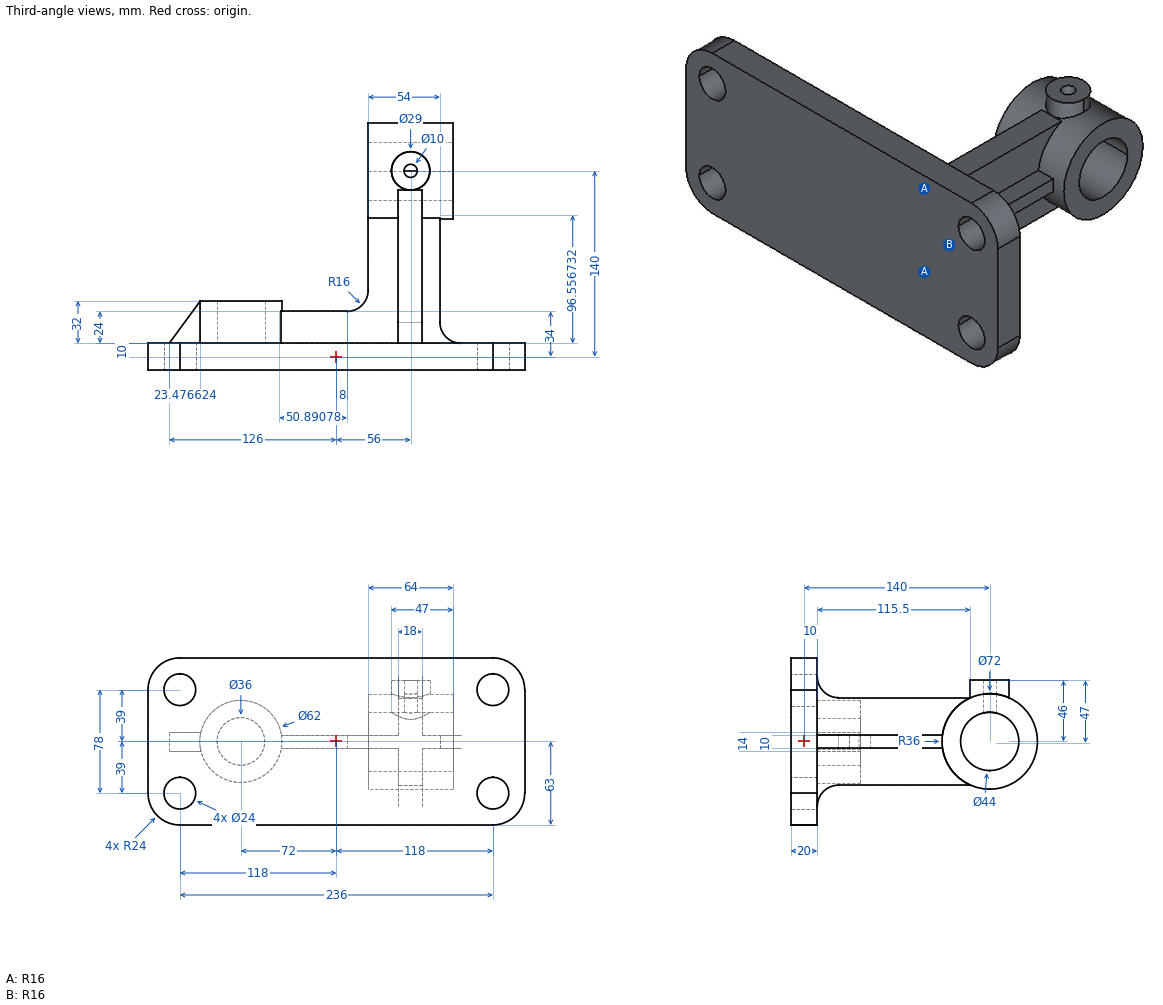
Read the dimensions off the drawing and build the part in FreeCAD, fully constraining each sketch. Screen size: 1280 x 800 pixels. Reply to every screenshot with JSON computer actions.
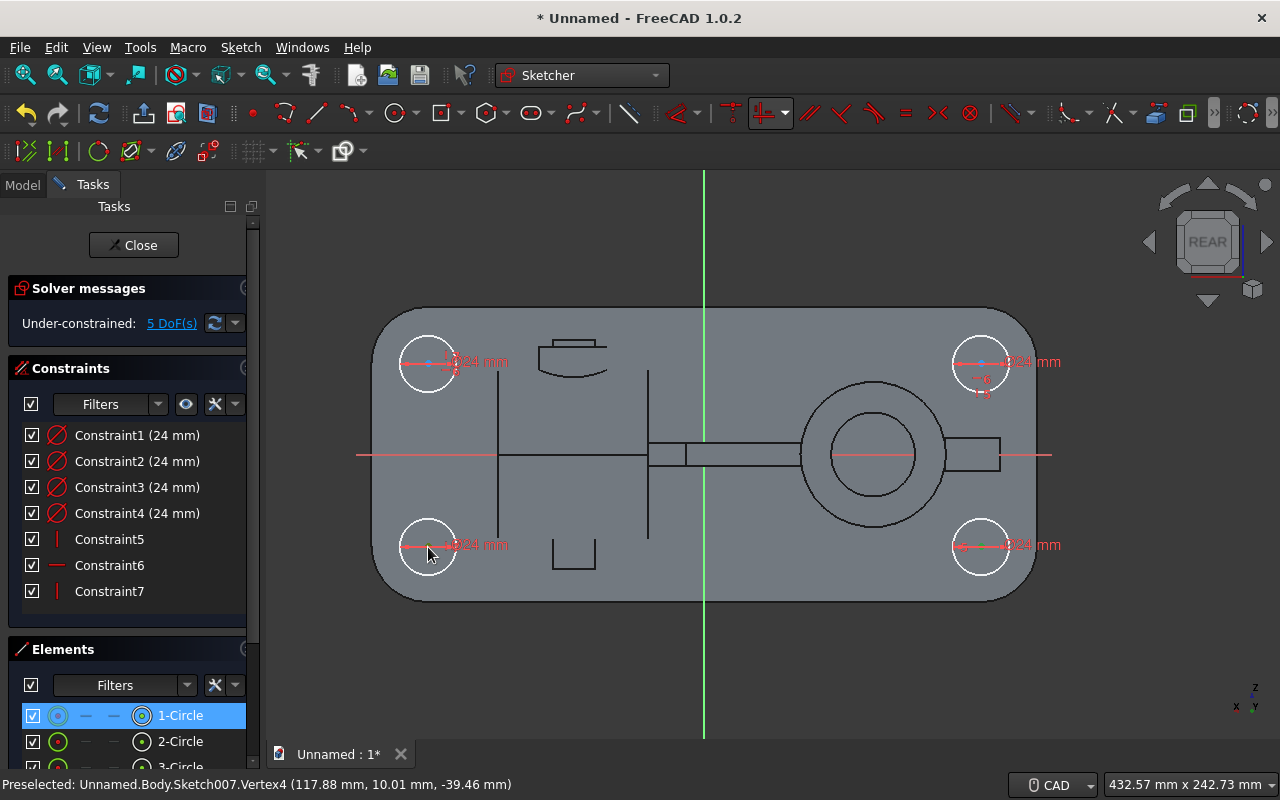
{"action": "key", "text": "h"}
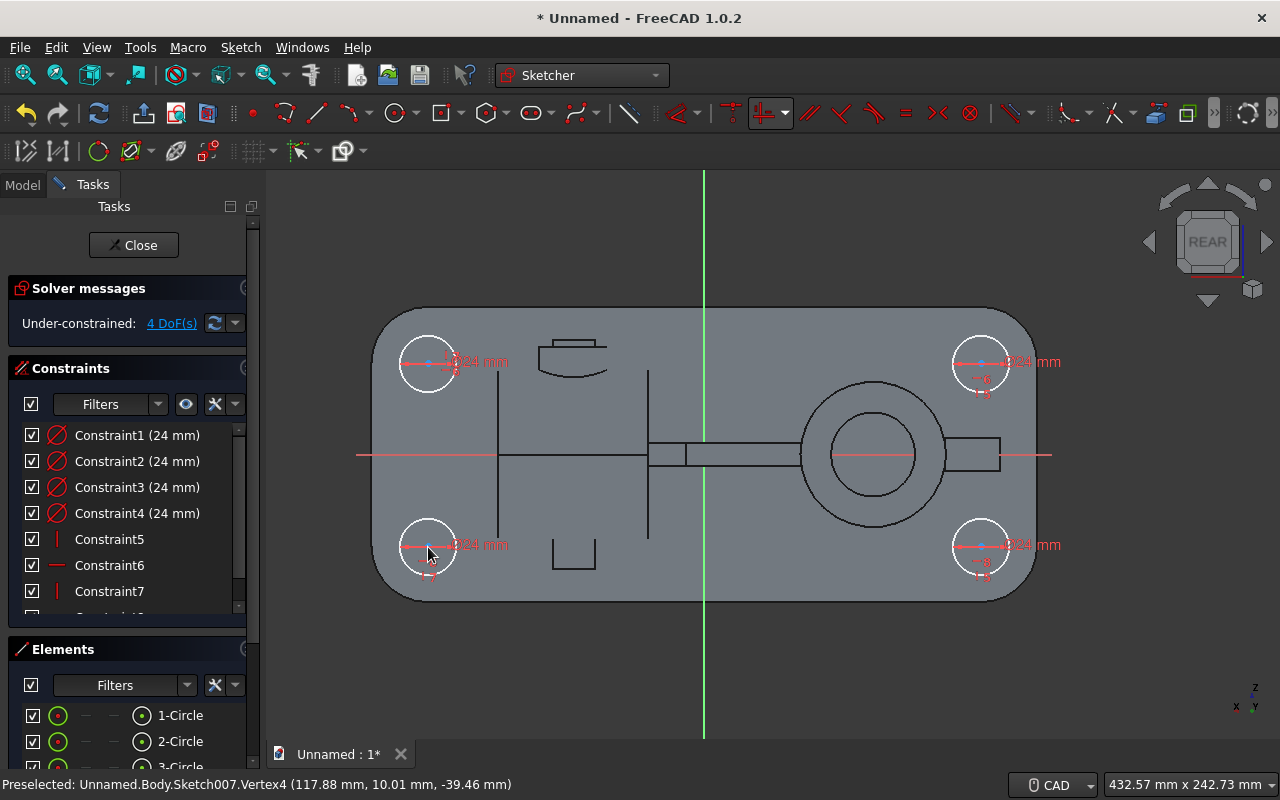
{"action": "left_click", "coordinate": [676, 114]}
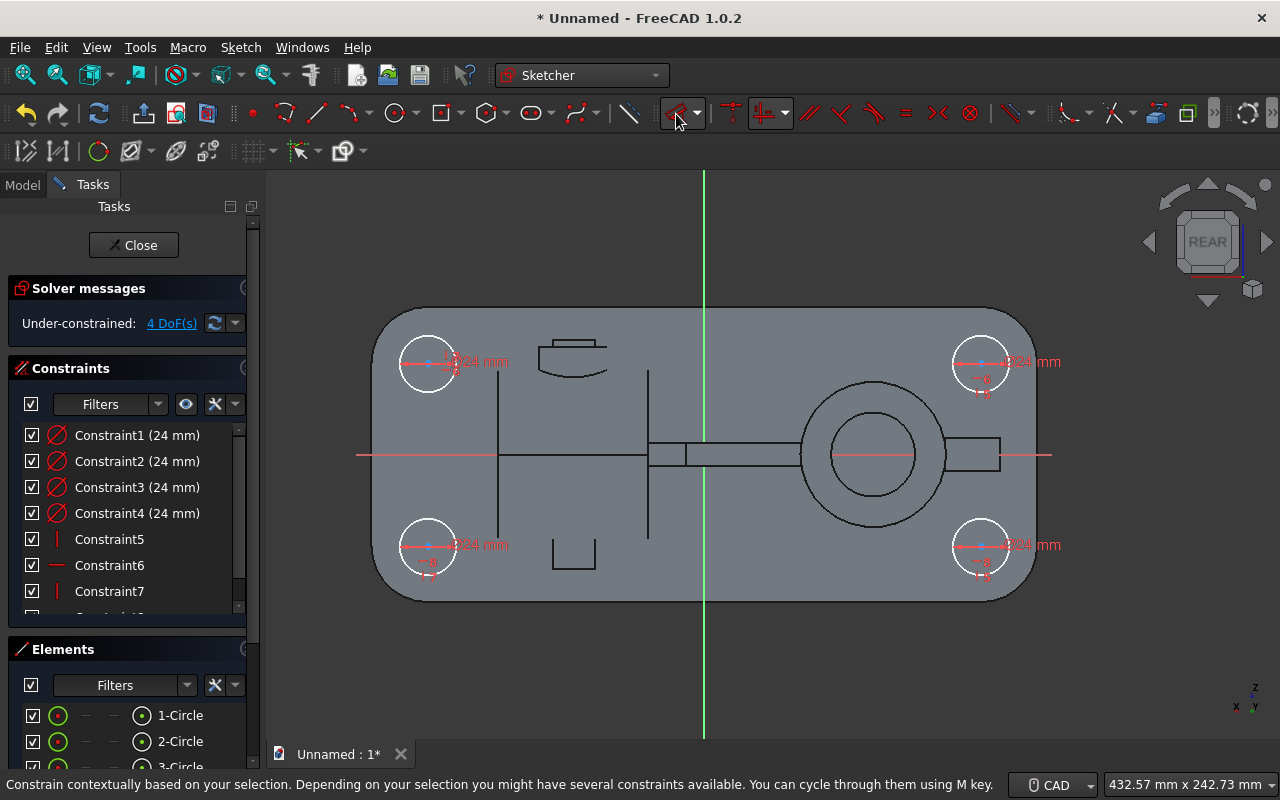
{"action": "left_click", "coordinate": [981, 547]}
{"action": "left_click", "coordinate": [1015, 501]}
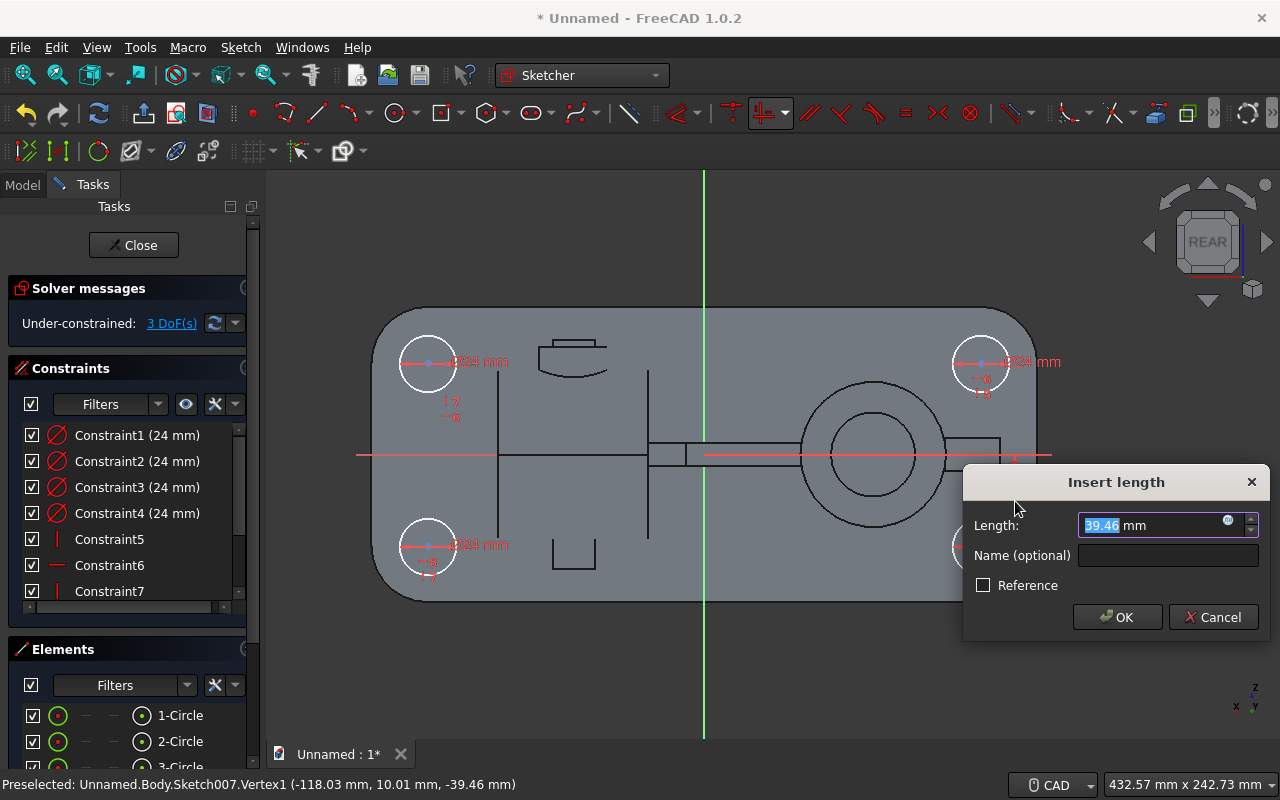
{"action": "type", "text": "39"}
{"action": "key", "text": "Return"}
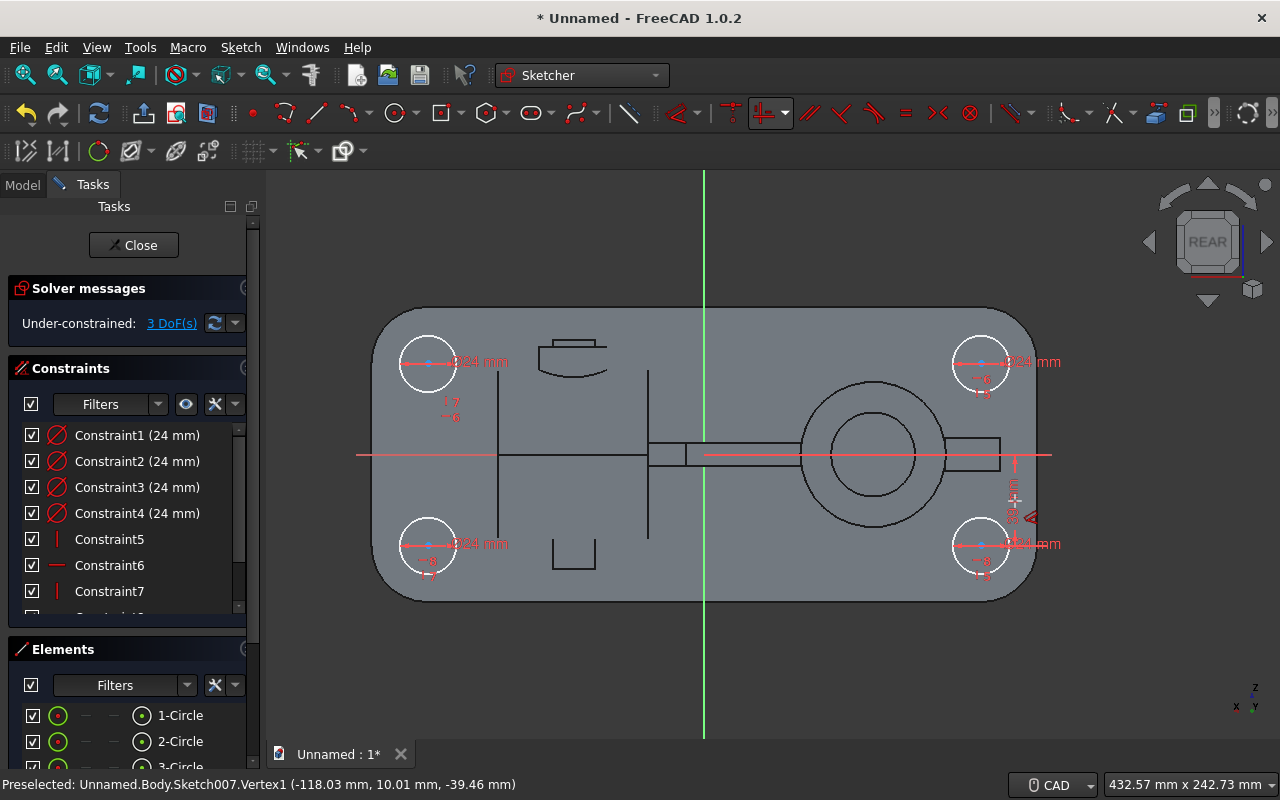
{"action": "left_click", "coordinate": [981, 364]}
{"action": "left_click", "coordinate": [1015, 409]}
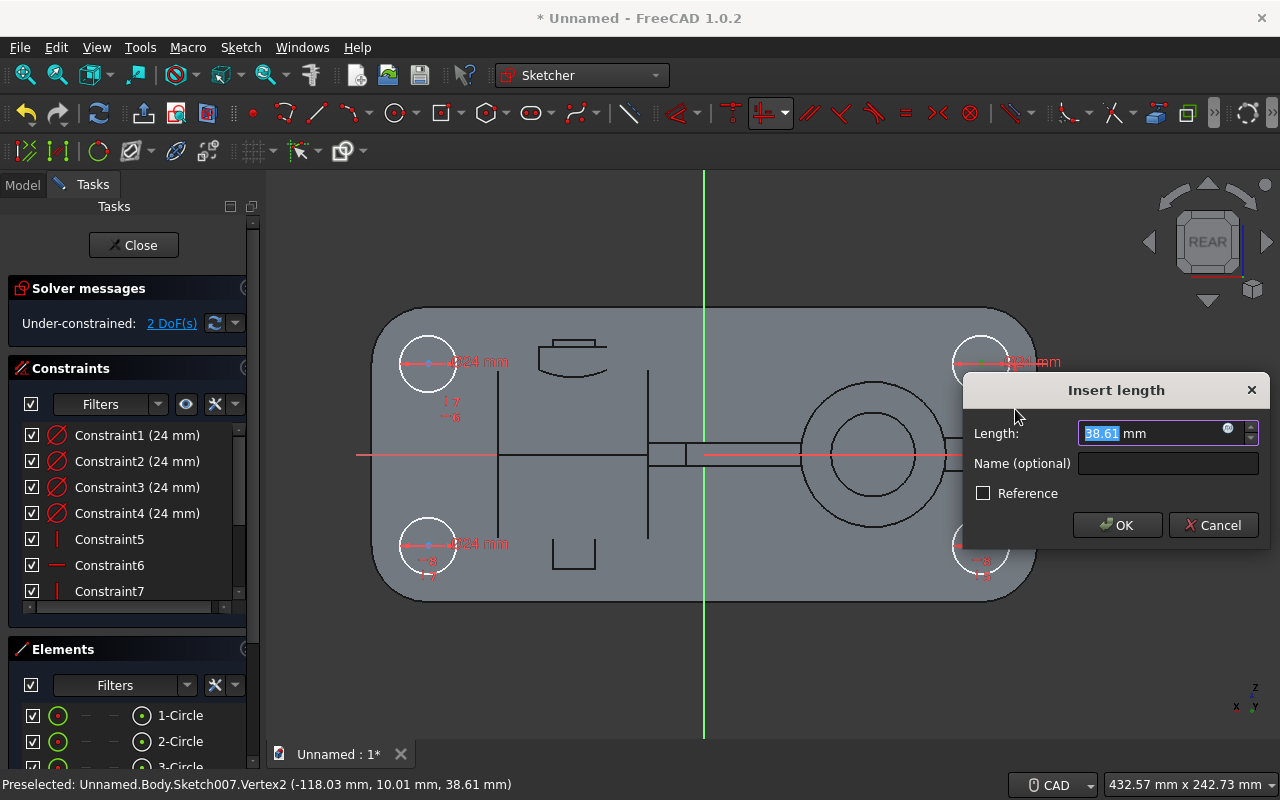
{"action": "type", "text": "39"}
{"action": "key", "text": "Return"}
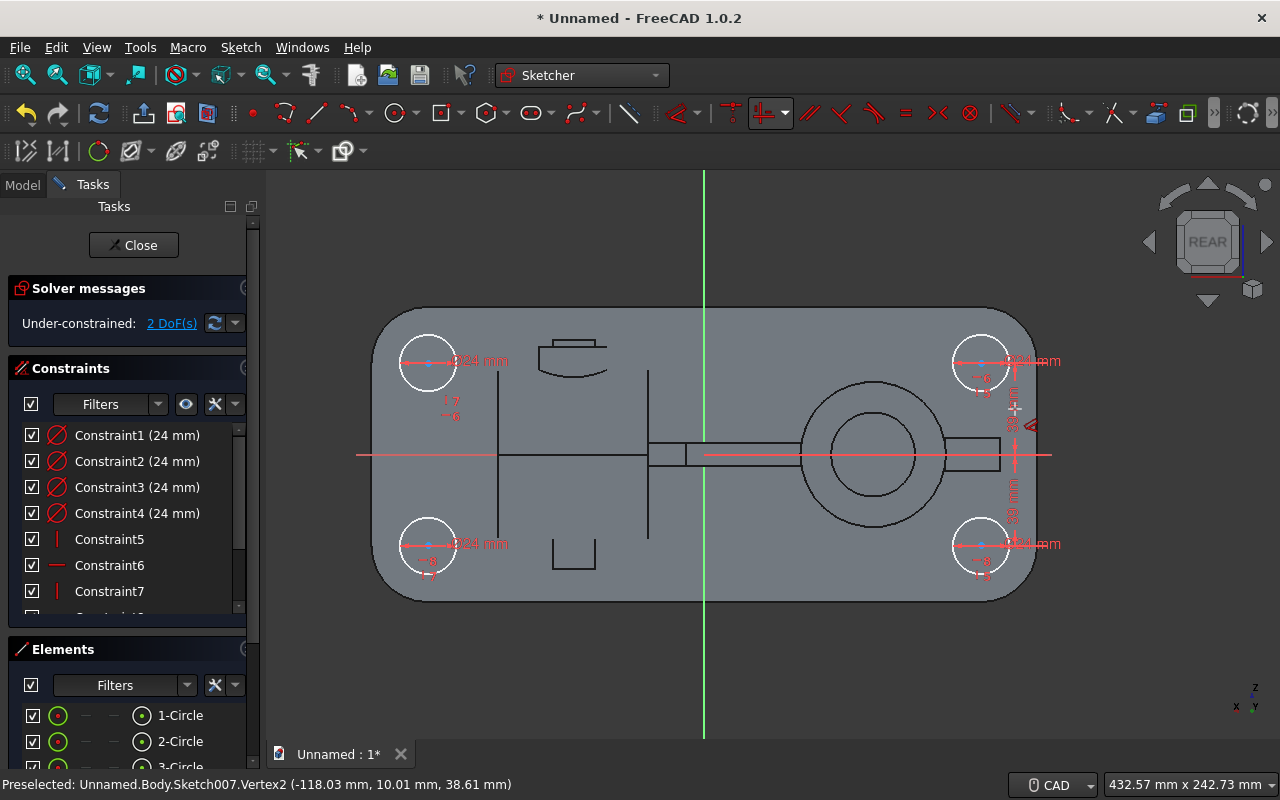
{"action": "left_click", "coordinate": [981, 546]}
{"action": "left_click", "coordinate": [843, 580]}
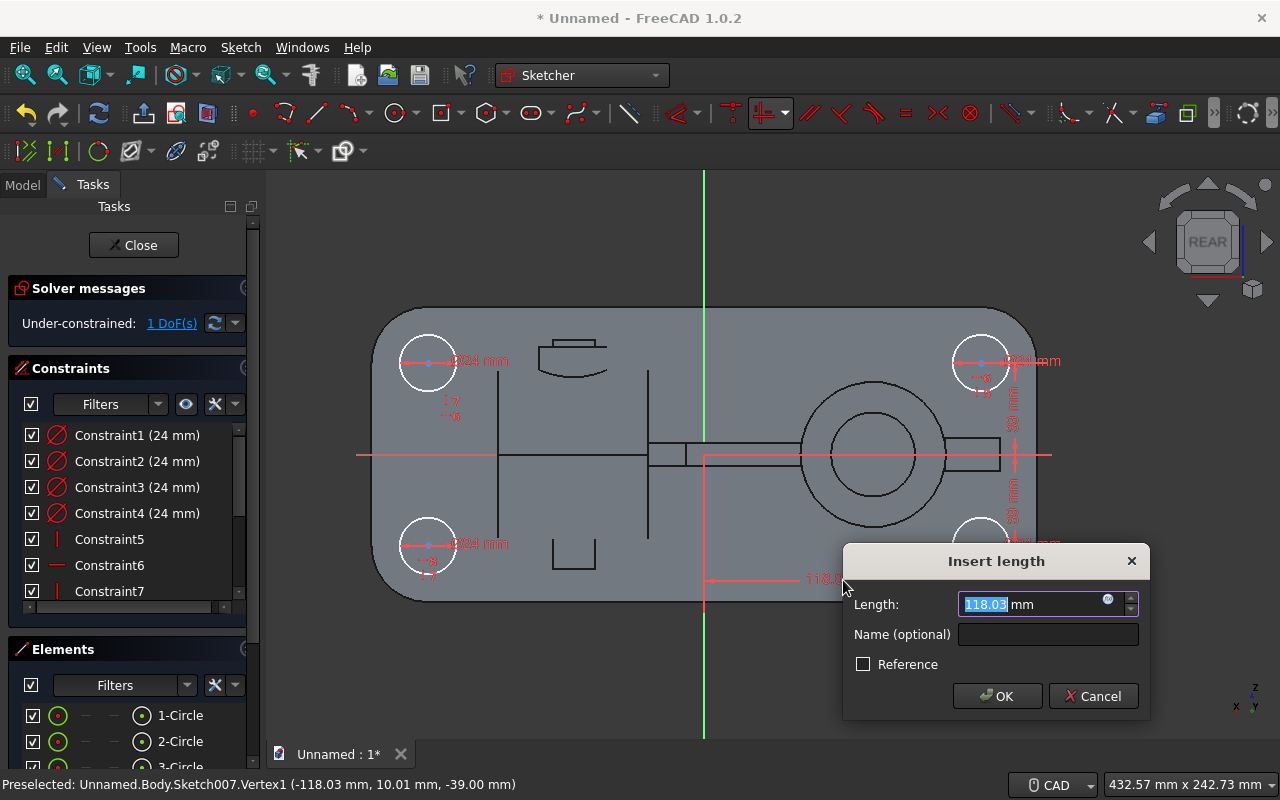
{"action": "type", "text": "118"}
{"action": "key", "text": "Return"}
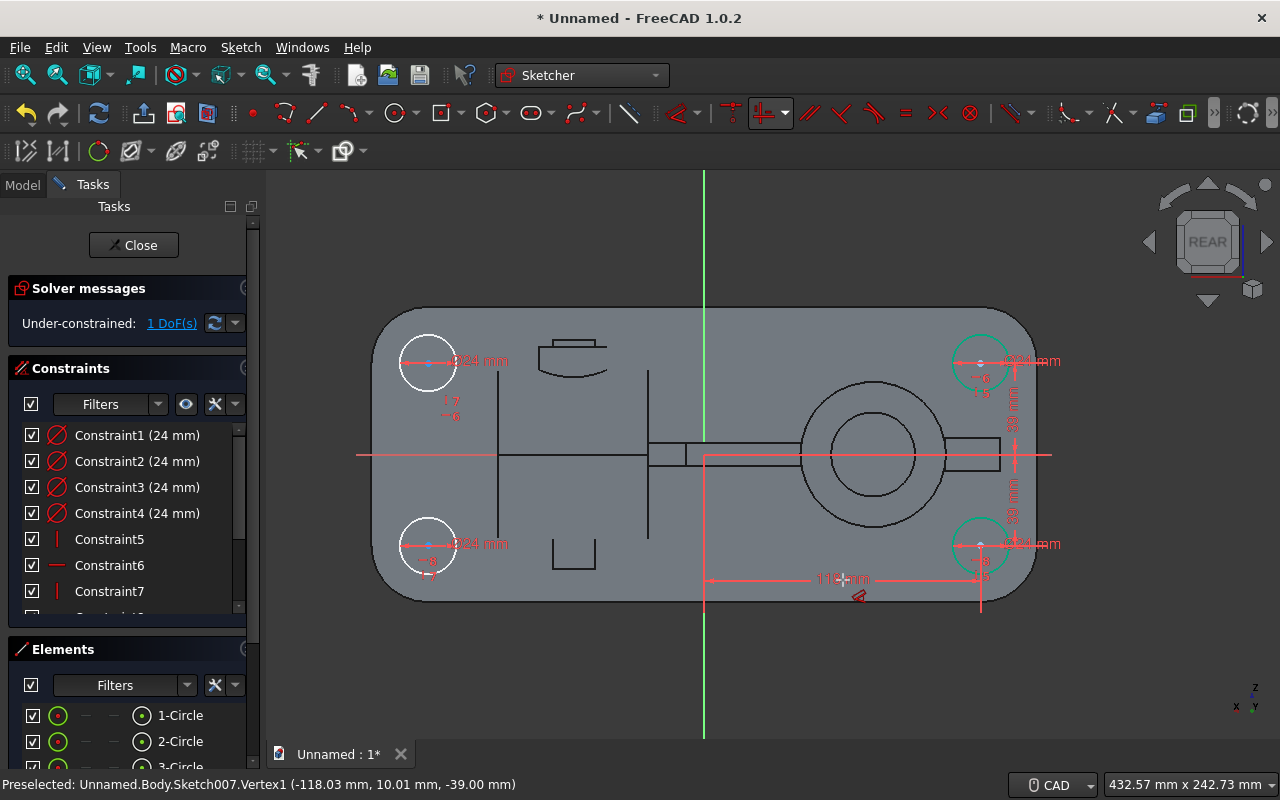
{"action": "left_click", "coordinate": [428, 363]}
{"action": "left_click", "coordinate": [566, 329]}